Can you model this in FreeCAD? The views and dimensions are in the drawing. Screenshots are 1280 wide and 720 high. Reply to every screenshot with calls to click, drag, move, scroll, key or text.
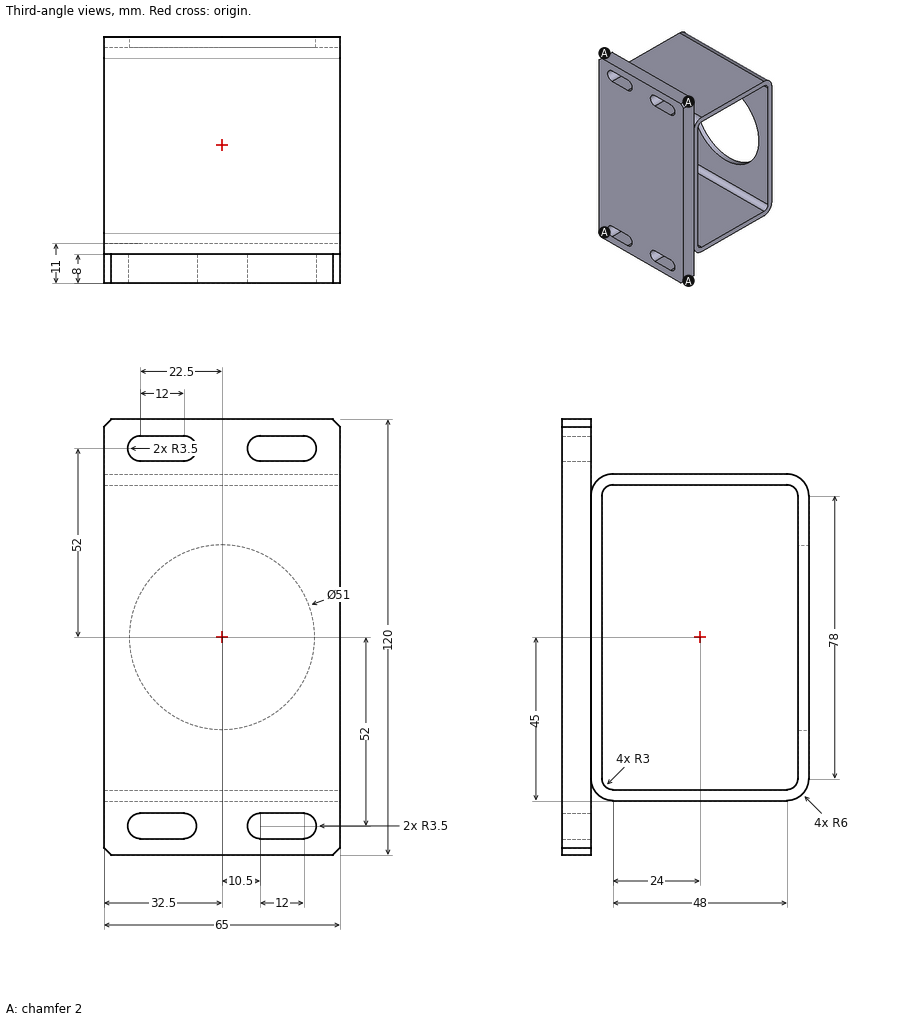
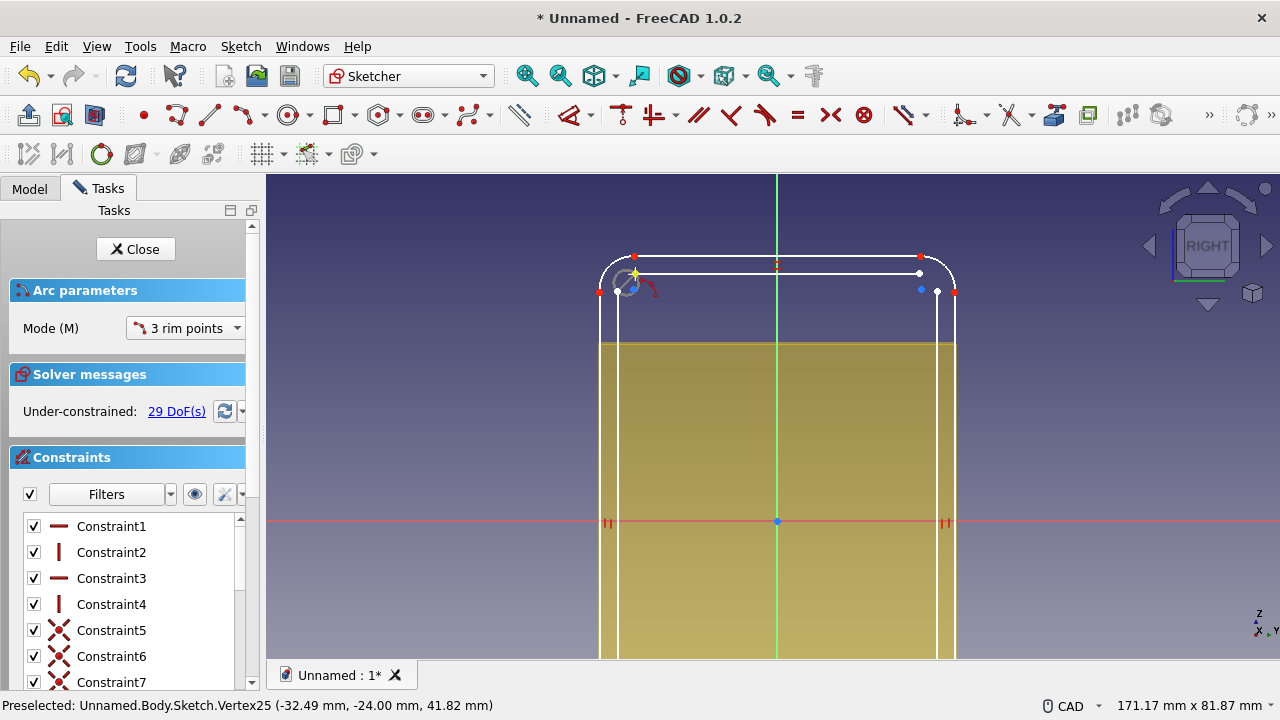
scroll(623, 278, up, 6)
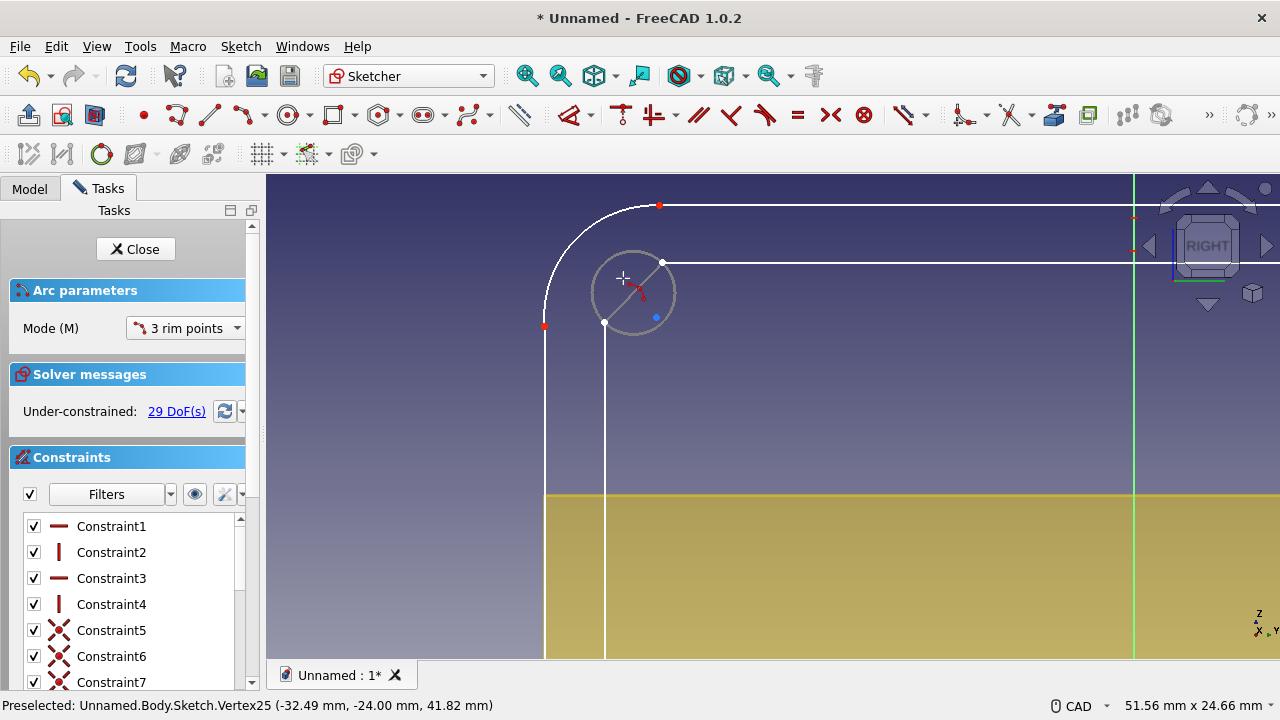
click(621, 277)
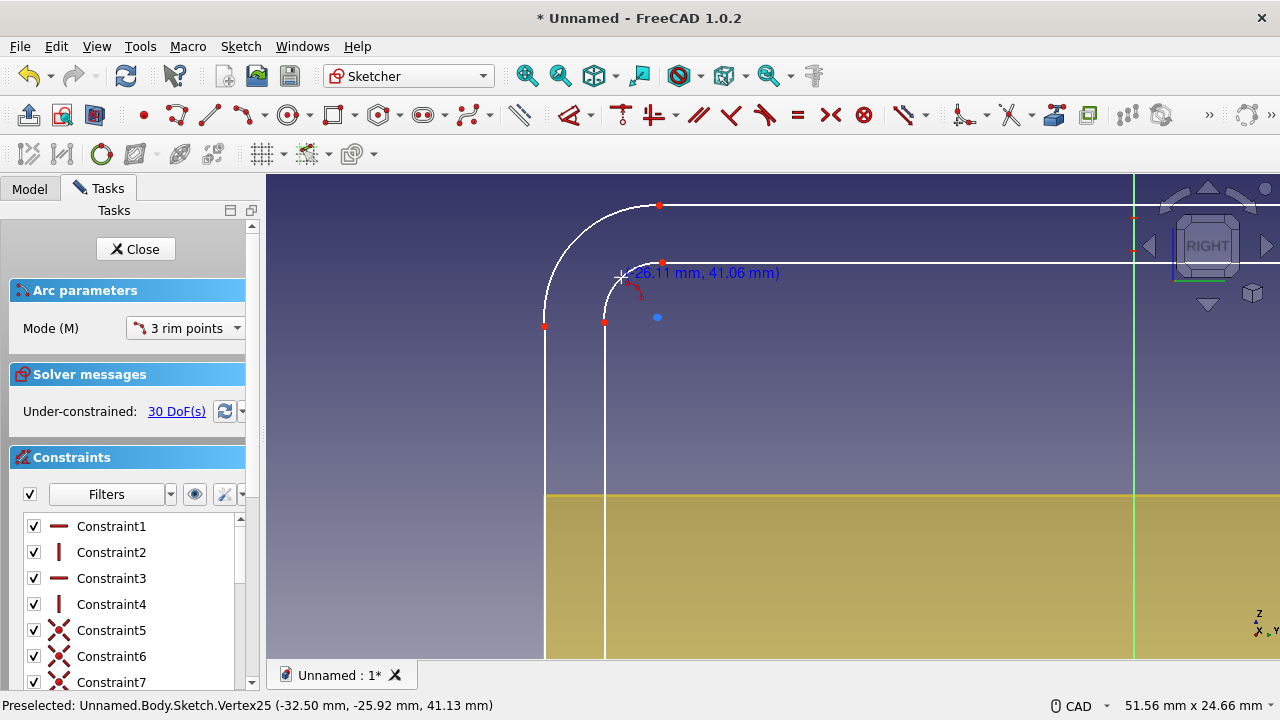
scroll(619, 284, down, 9)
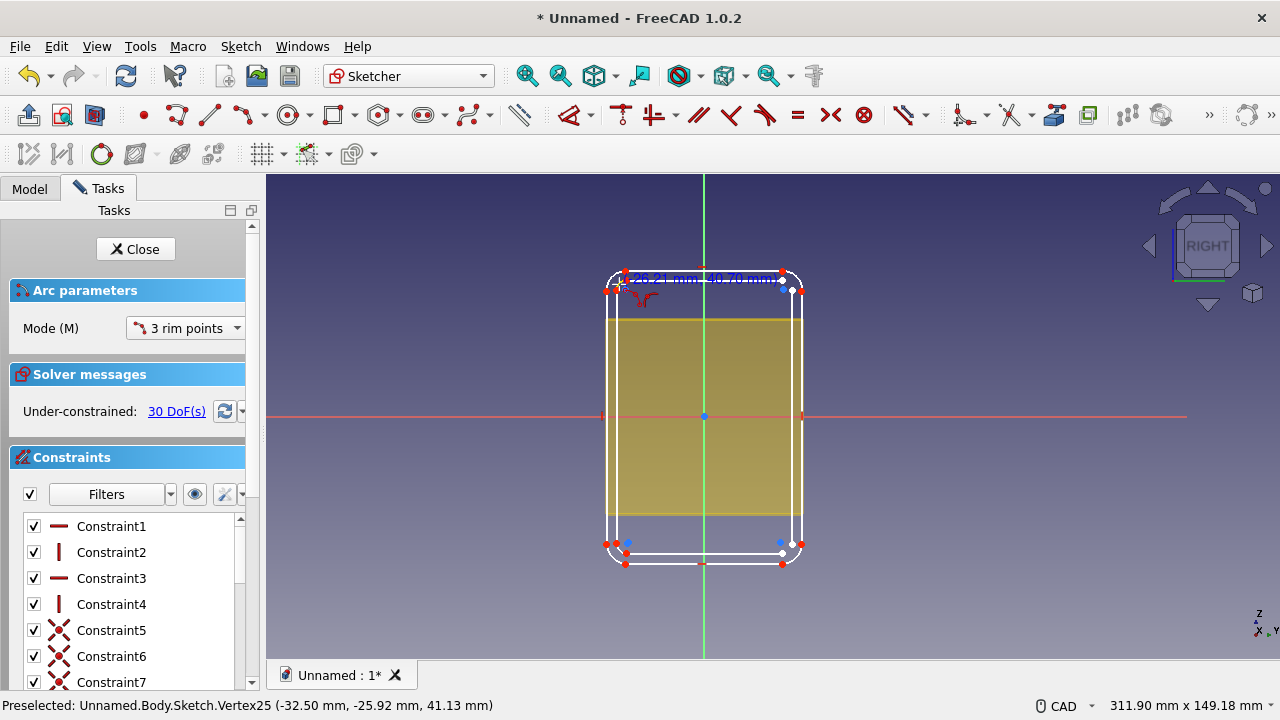
scroll(783, 280, up, 3)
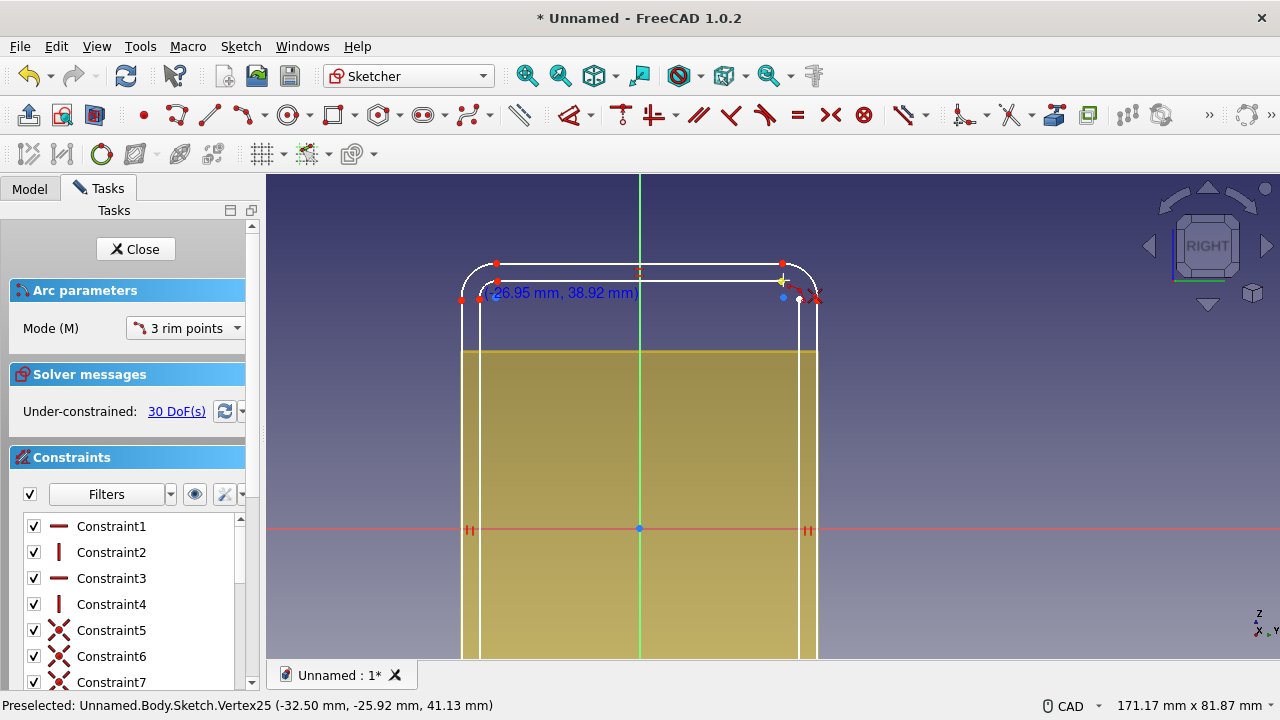
click(781, 281)
click(799, 299)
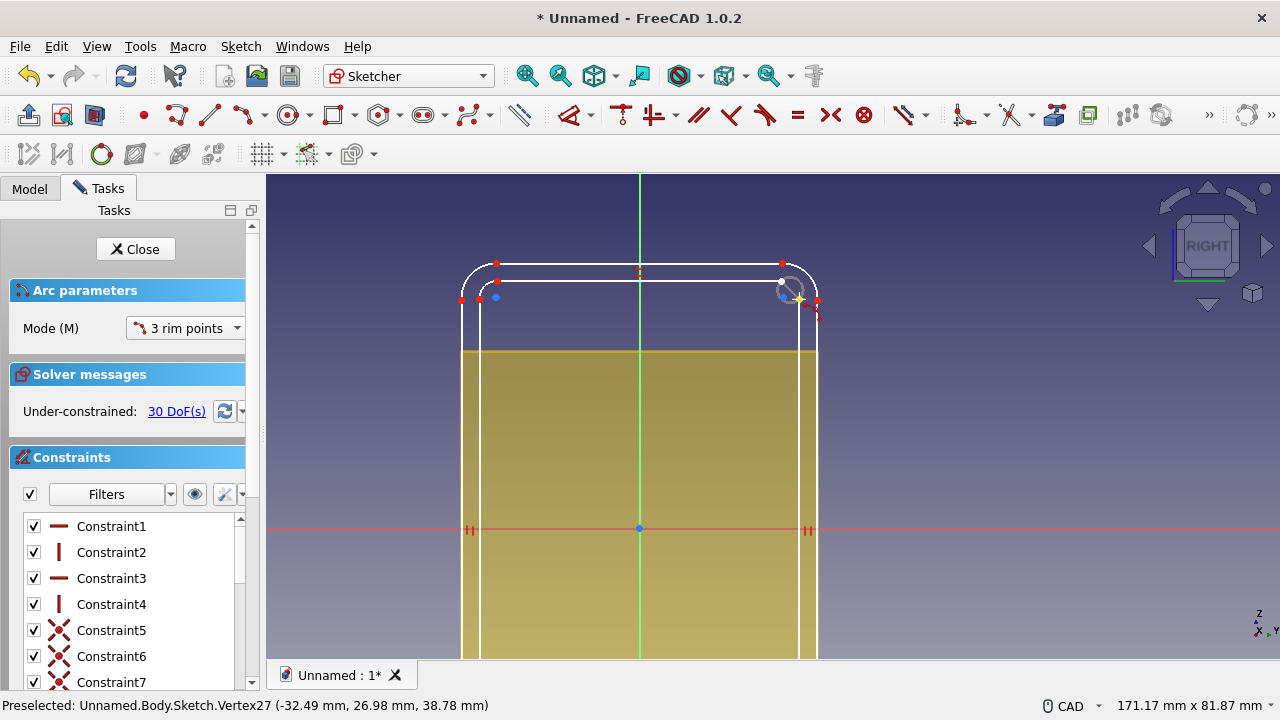
scroll(794, 285, up, 6)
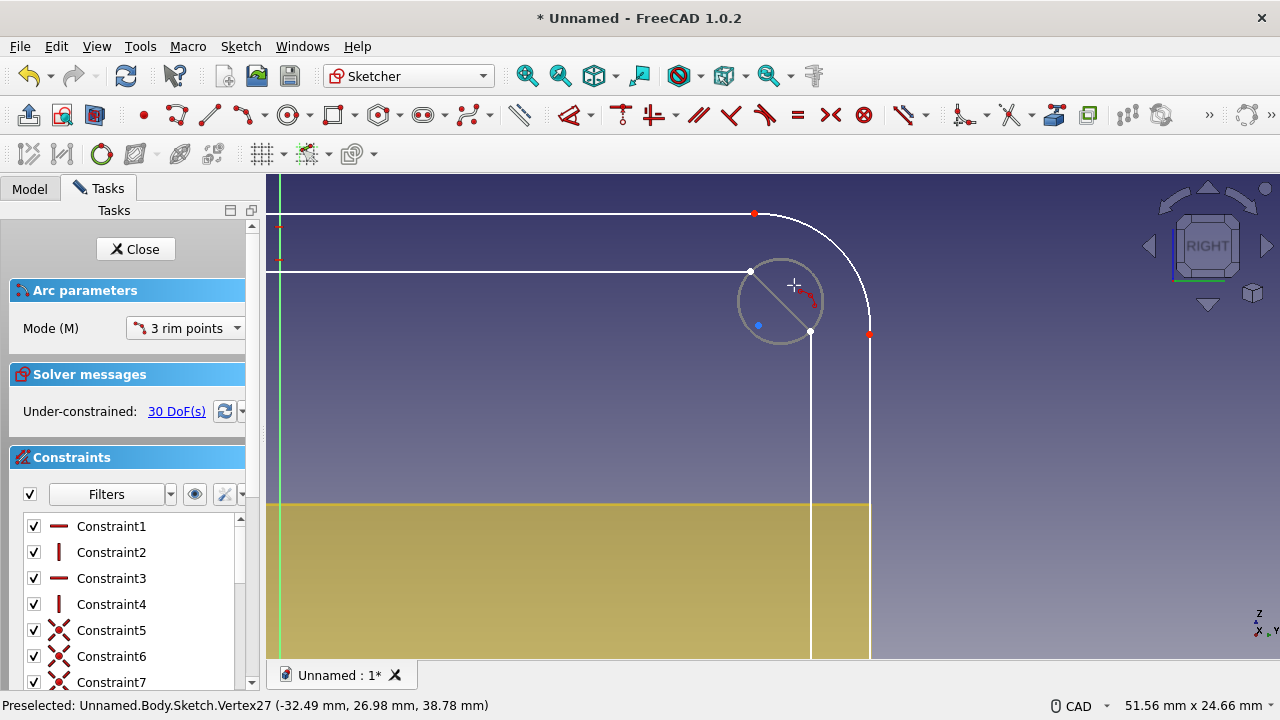
click(794, 285)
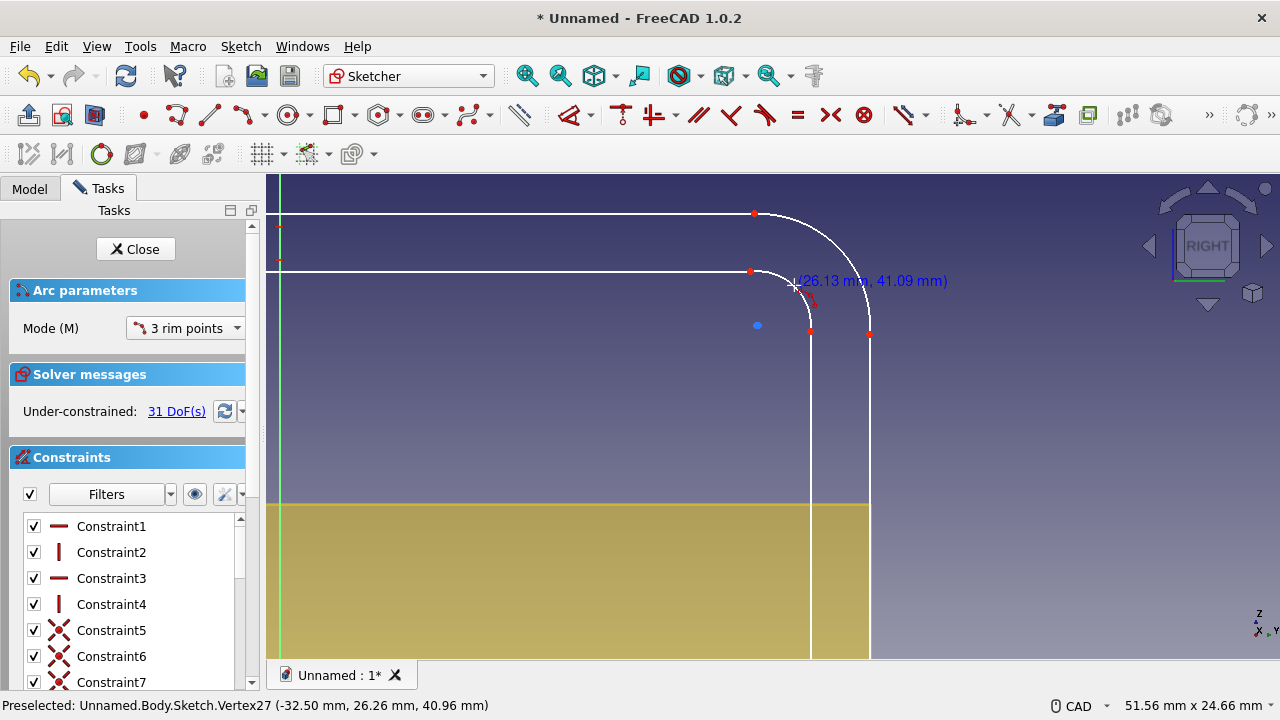
scroll(789, 282, down, 9)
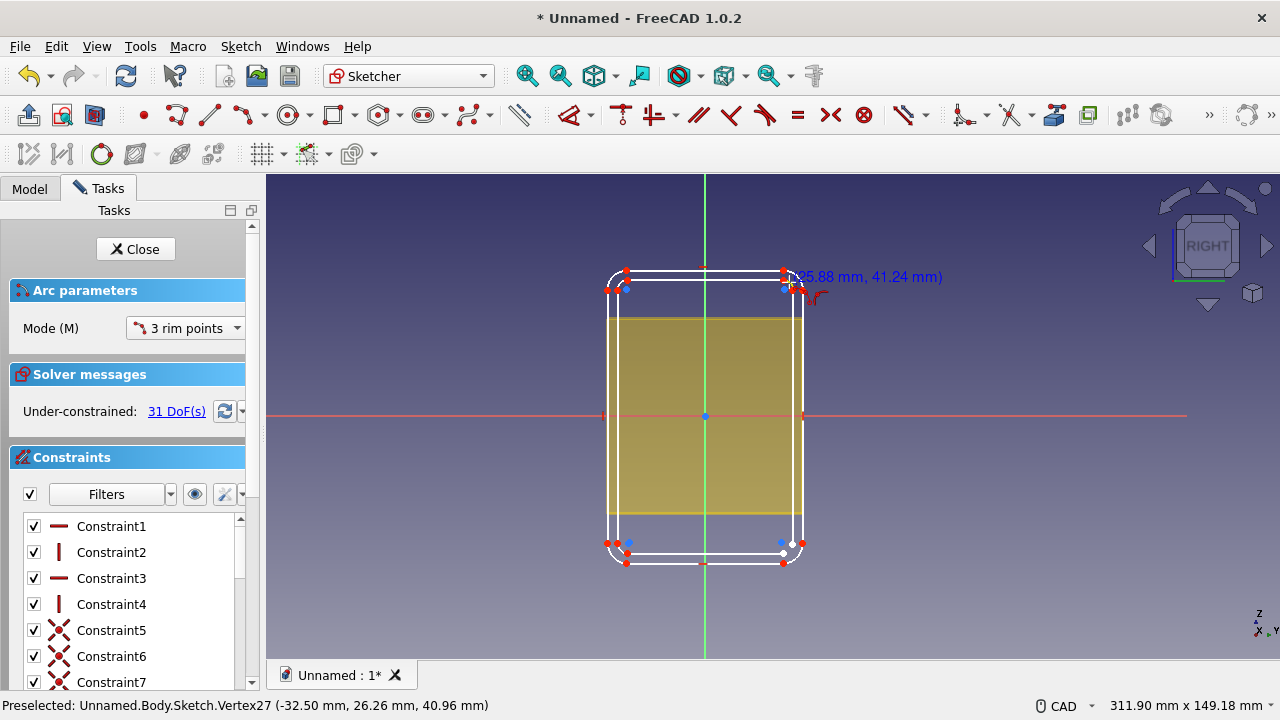
scroll(793, 543, up, 3)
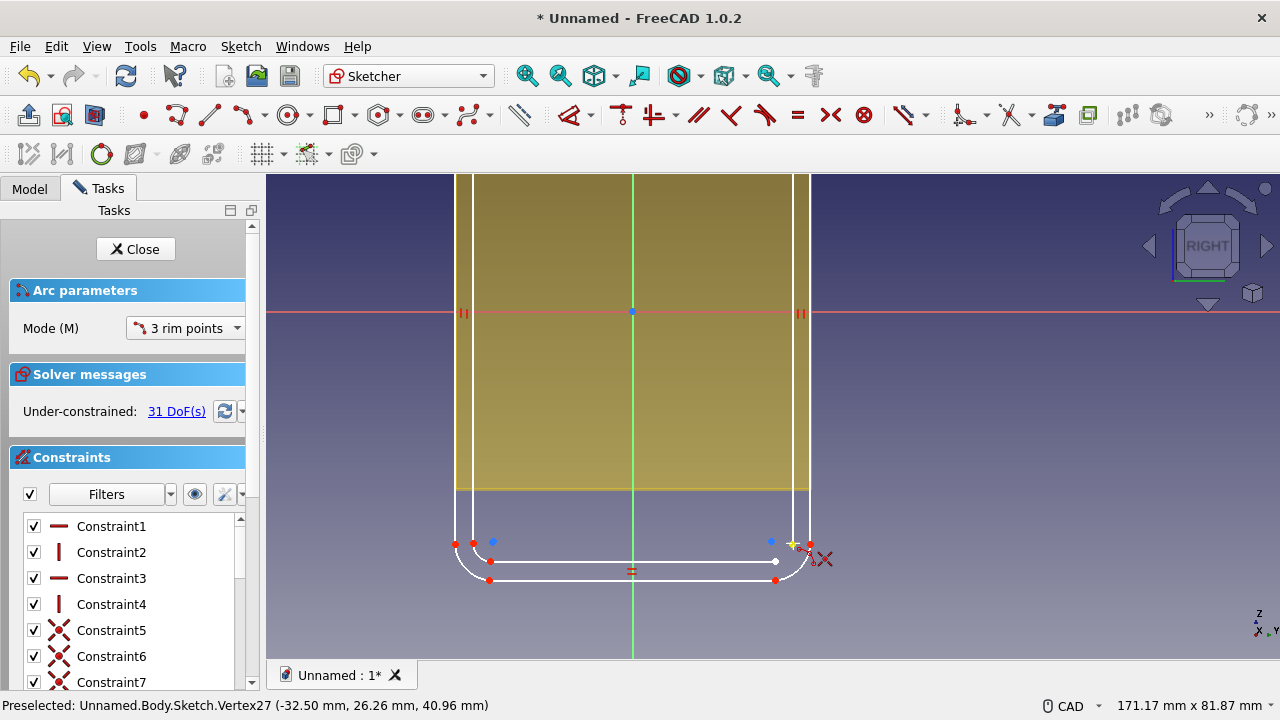
click(793, 544)
click(775, 562)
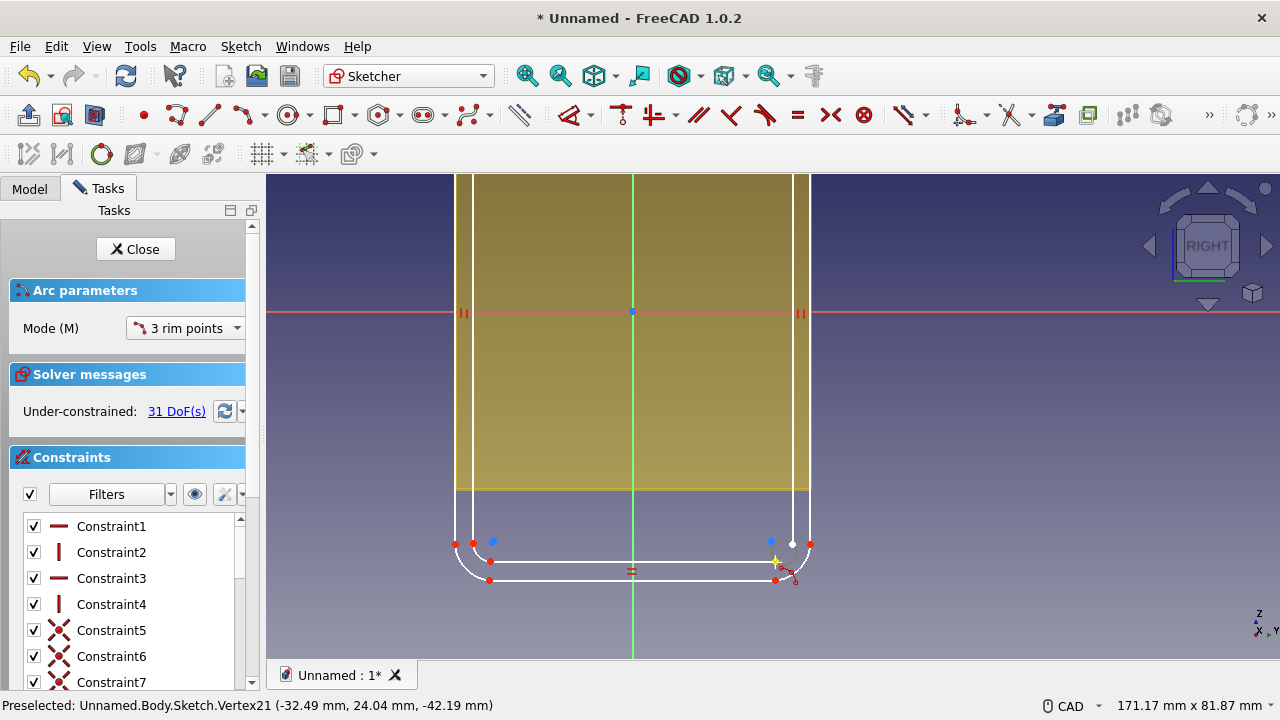
scroll(787, 555, up, 6)